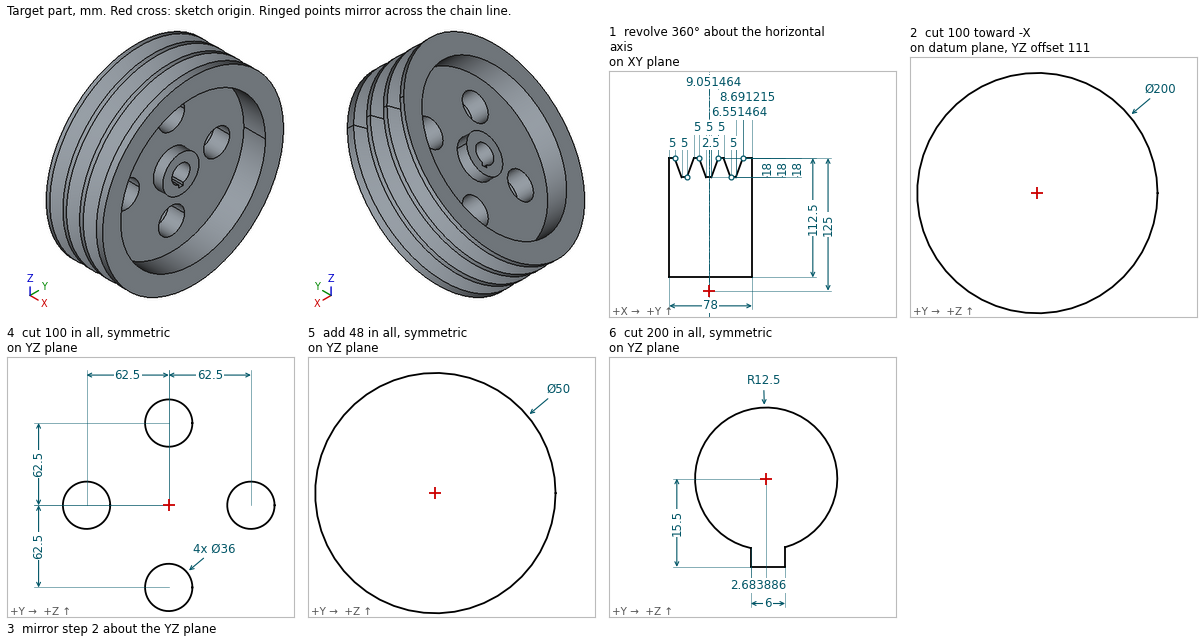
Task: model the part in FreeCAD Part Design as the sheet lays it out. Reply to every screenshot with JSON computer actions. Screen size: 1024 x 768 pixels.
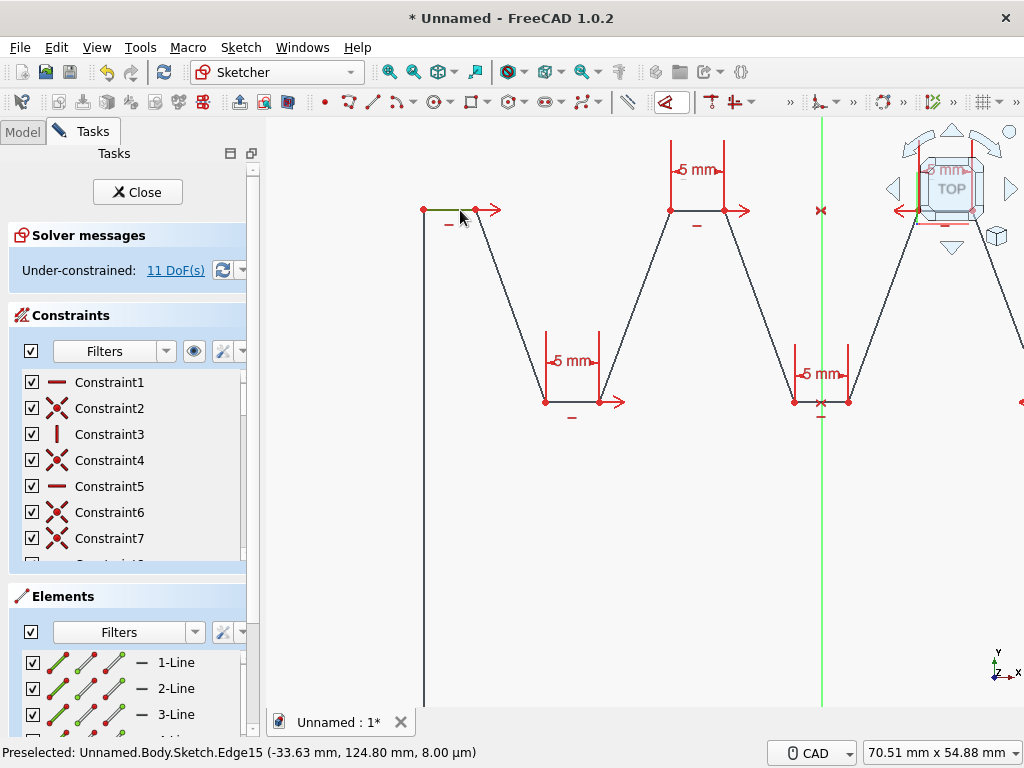
{"action": "left_click", "coordinate": [684, 102]}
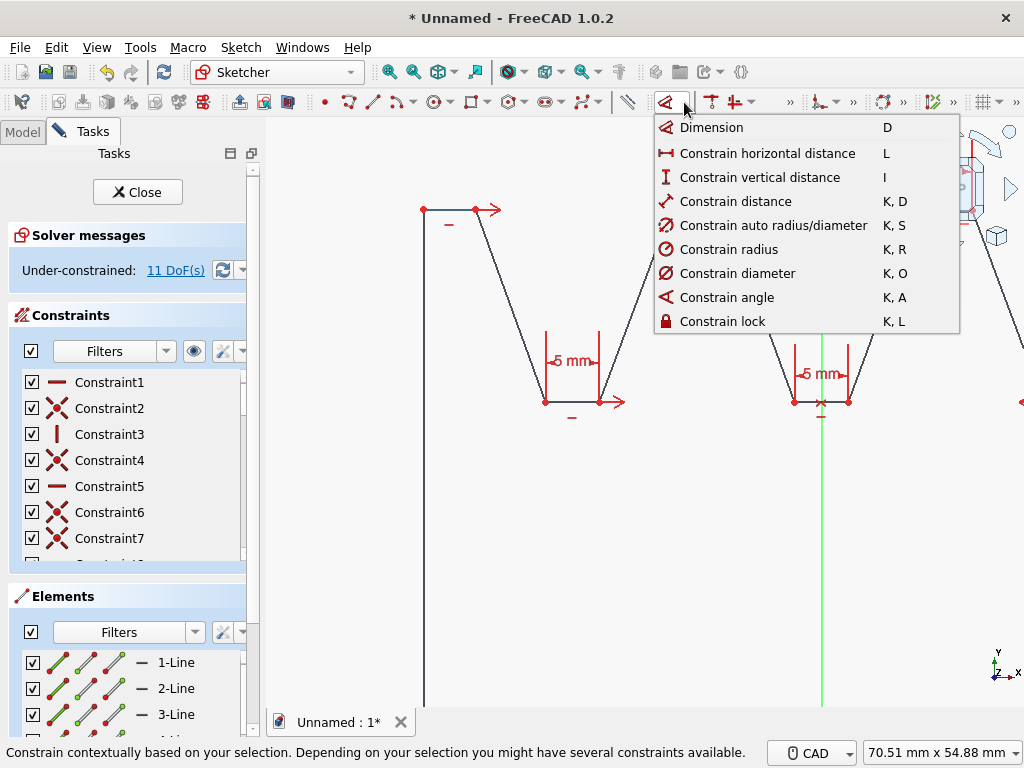
{"action": "left_click", "coordinate": [807, 153]}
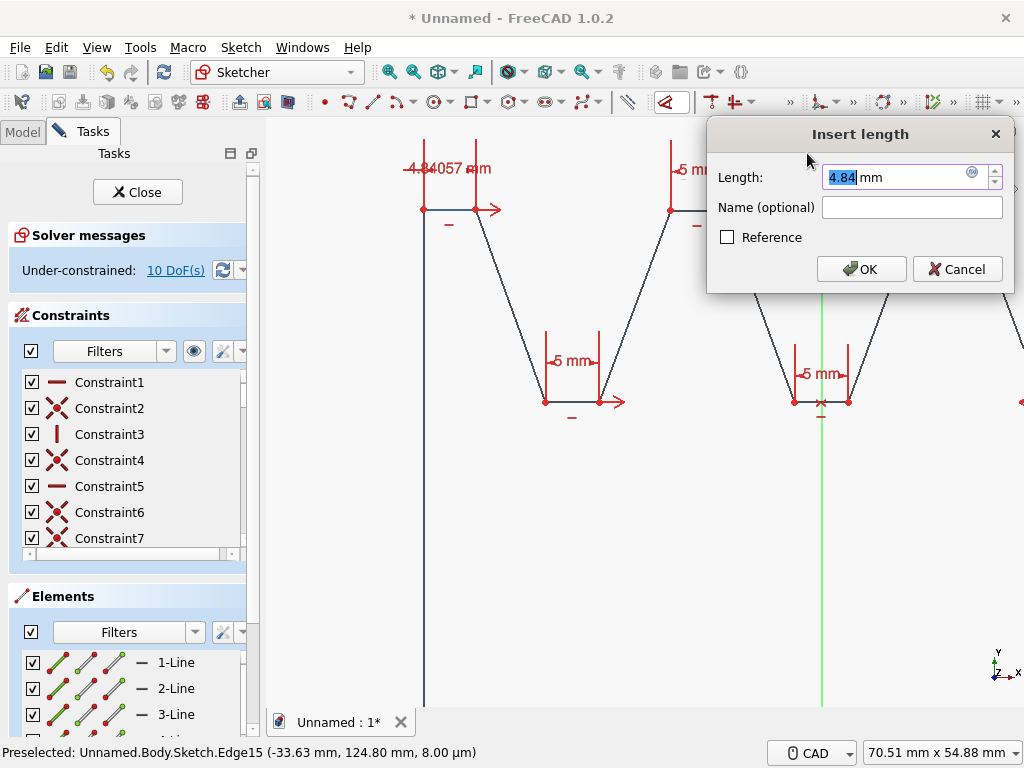
{"action": "type", "text": "5"}
{"action": "key", "text": "Return"}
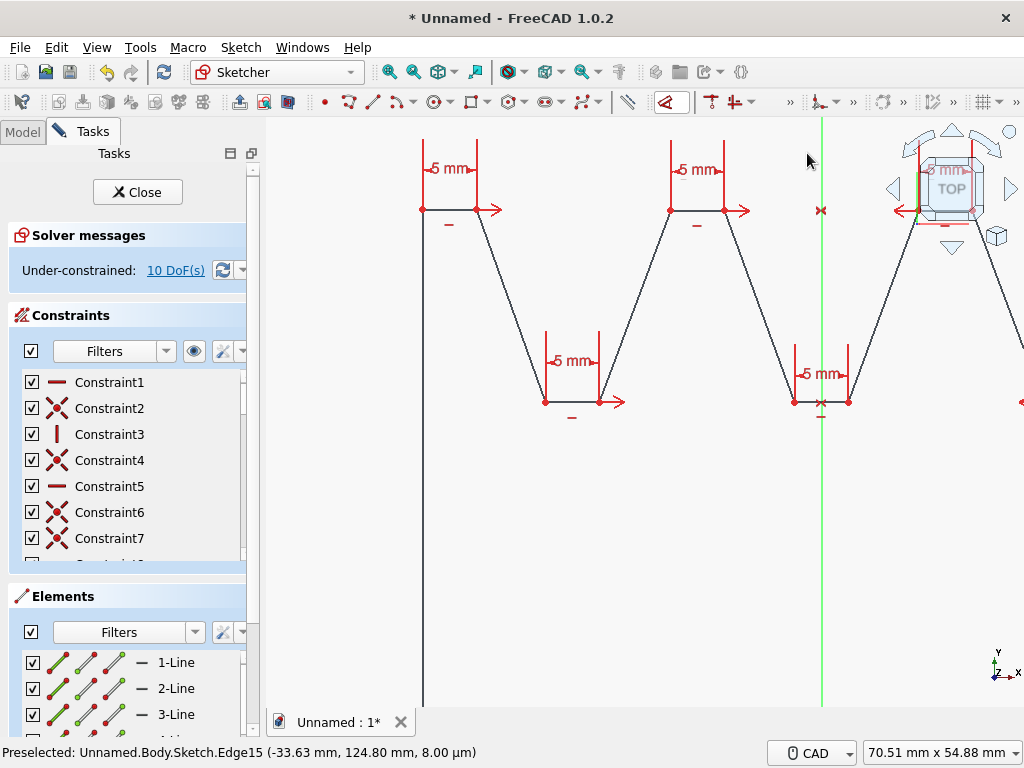
{"action": "scroll", "coordinate": [462, 210], "scroll_direction": "down", "scroll_amount": 6}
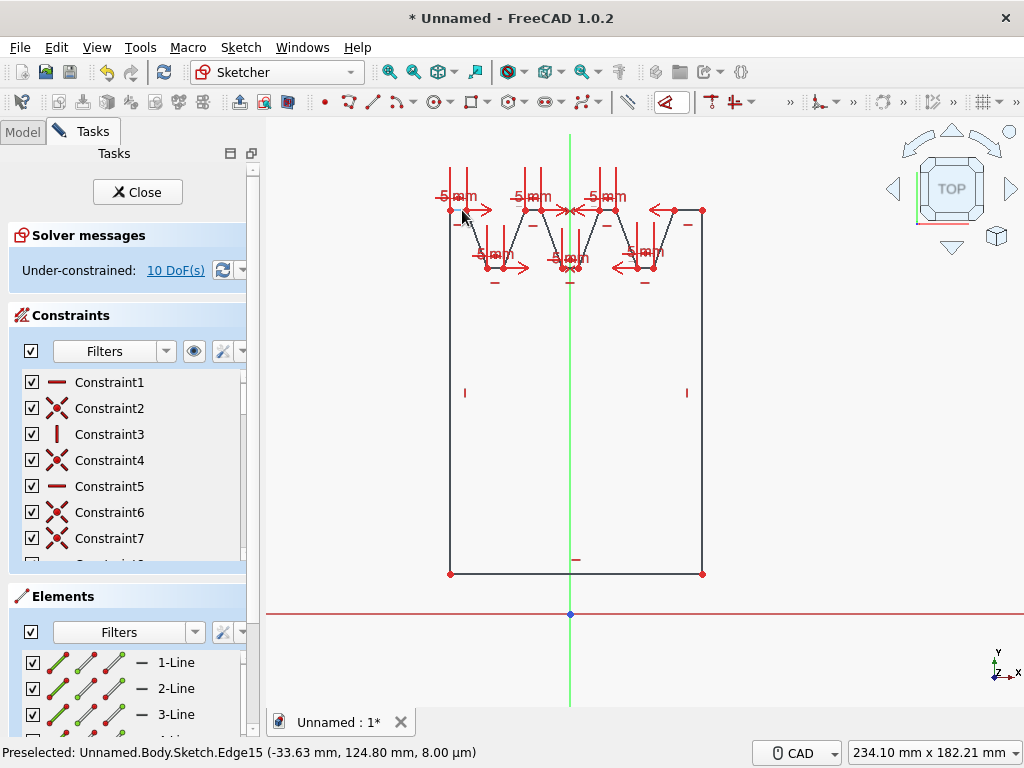
{"action": "left_click", "coordinate": [526, 574]}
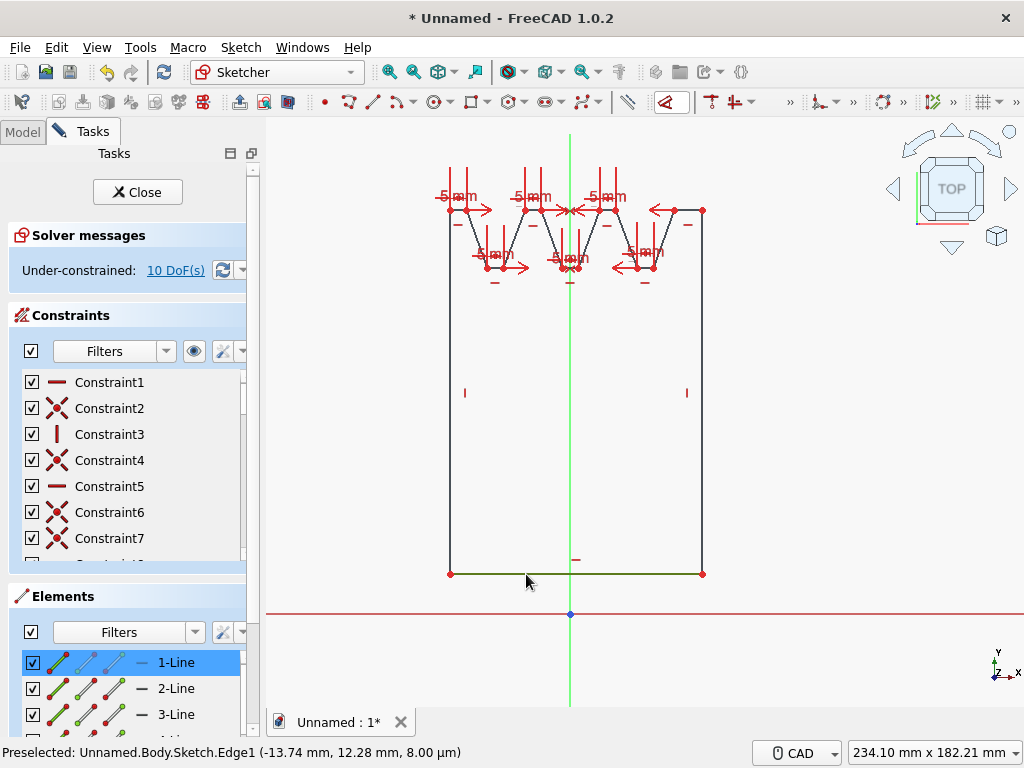
{"action": "key", "text": "l"}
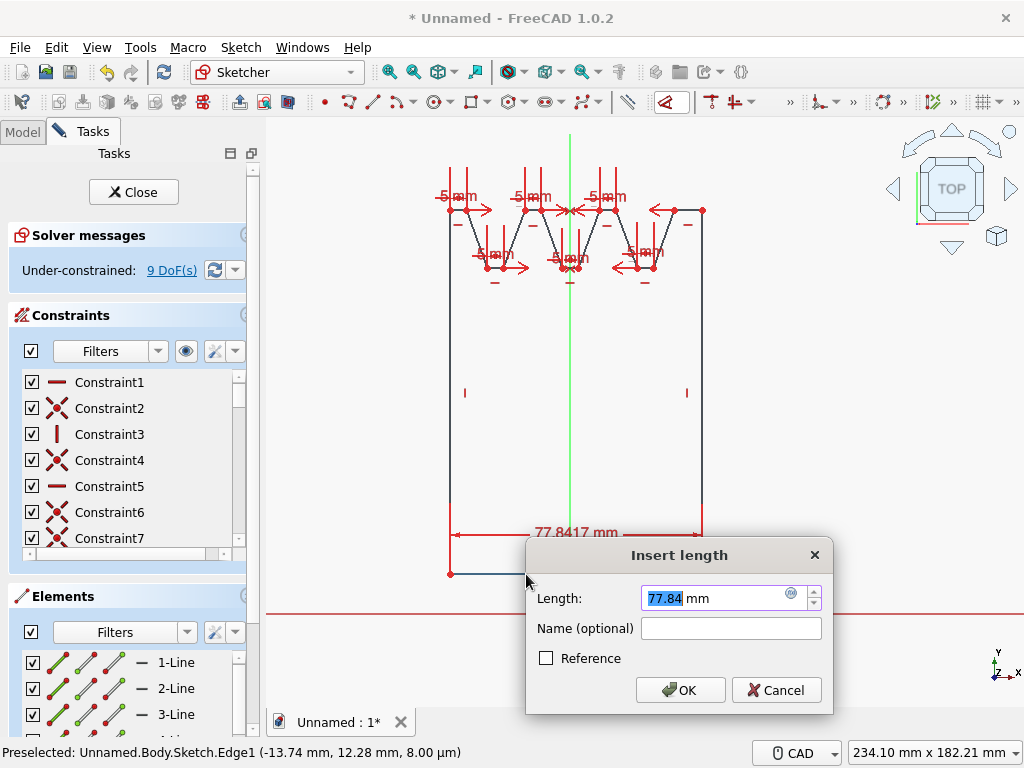
{"action": "type", "text": "78"}
{"action": "key", "text": "Return"}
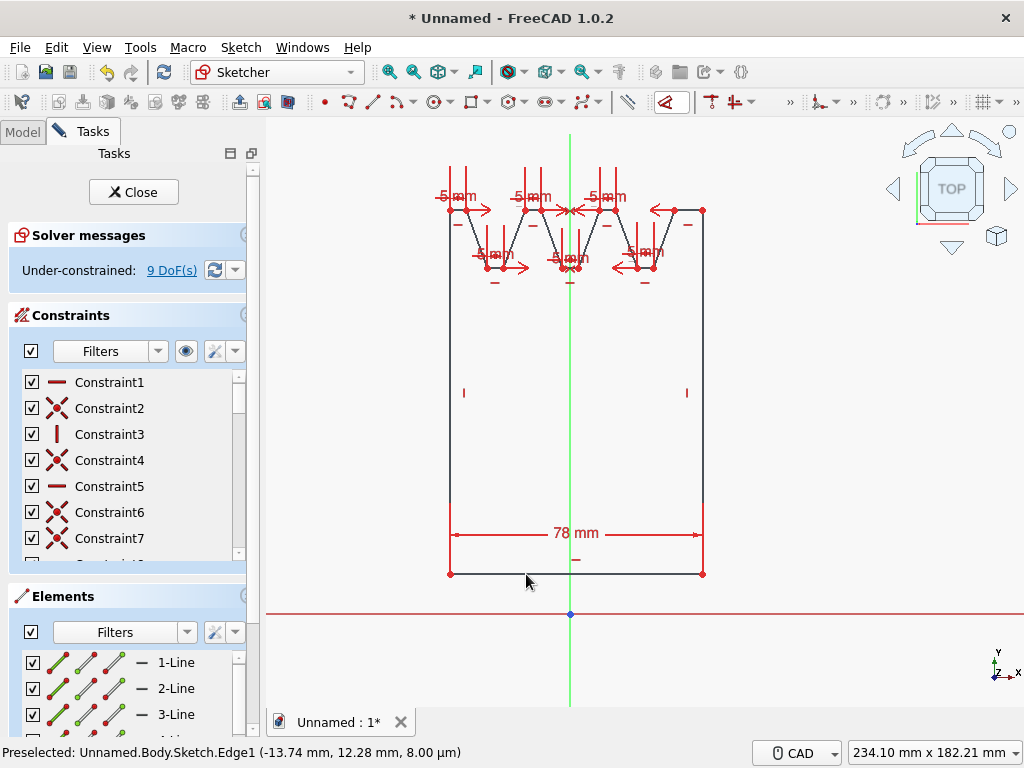
{"action": "left_click", "coordinate": [668, 227]}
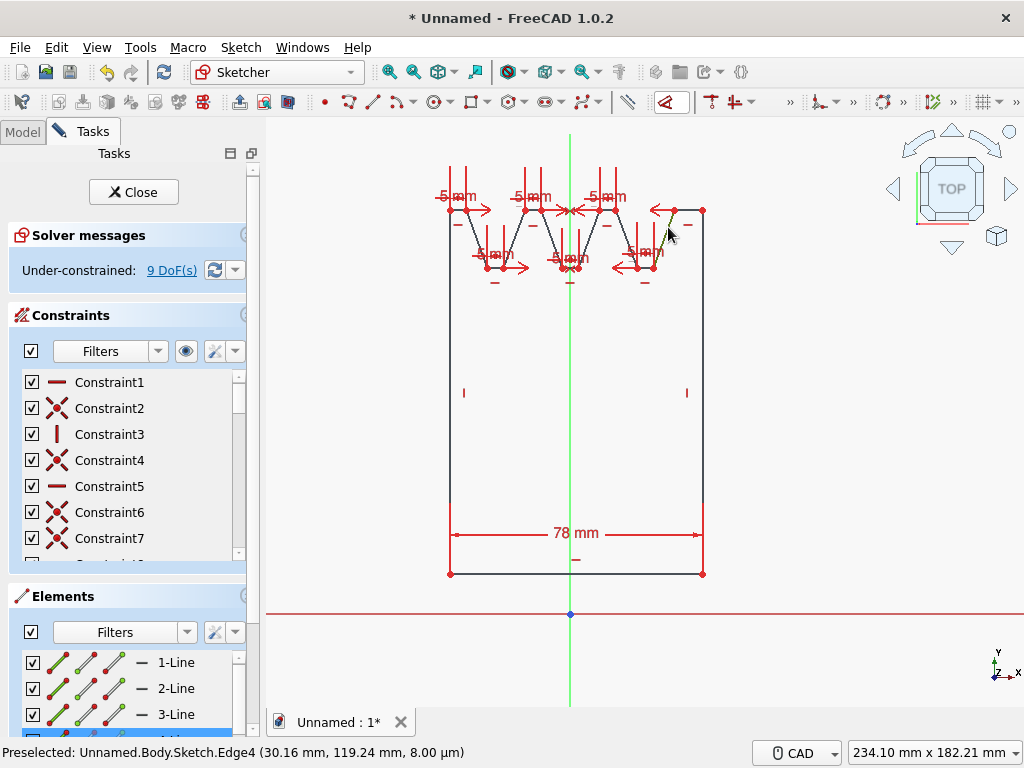
{"action": "key", "text": "i"}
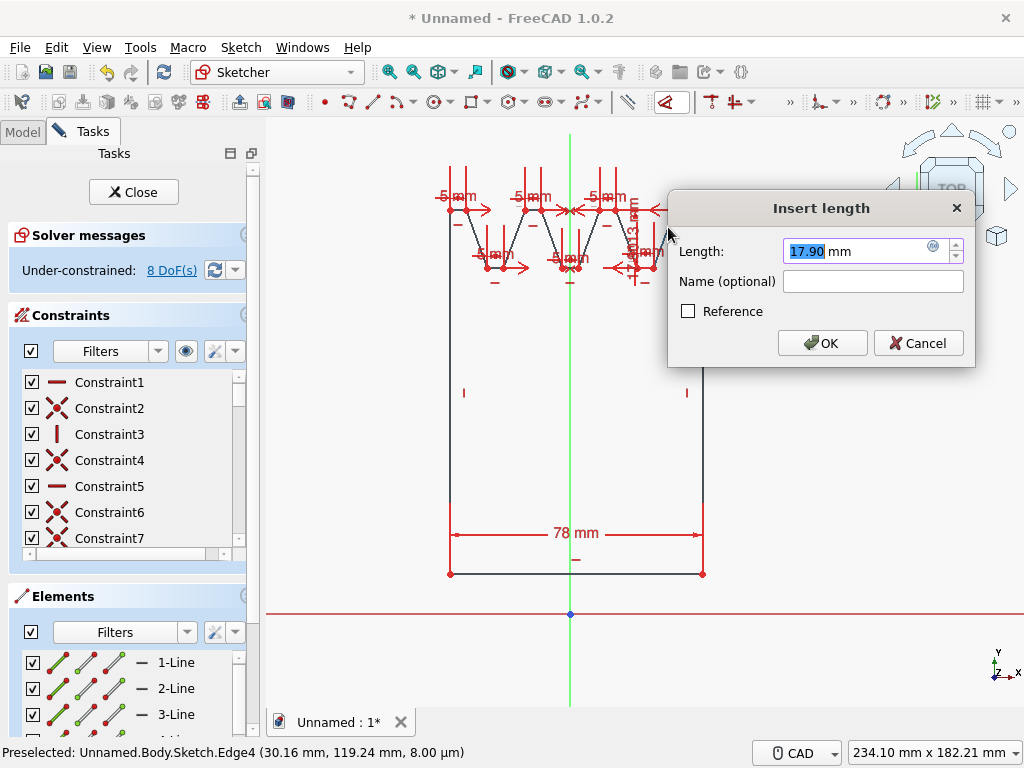
{"action": "type", "text": "18"}
{"action": "key", "text": "Return"}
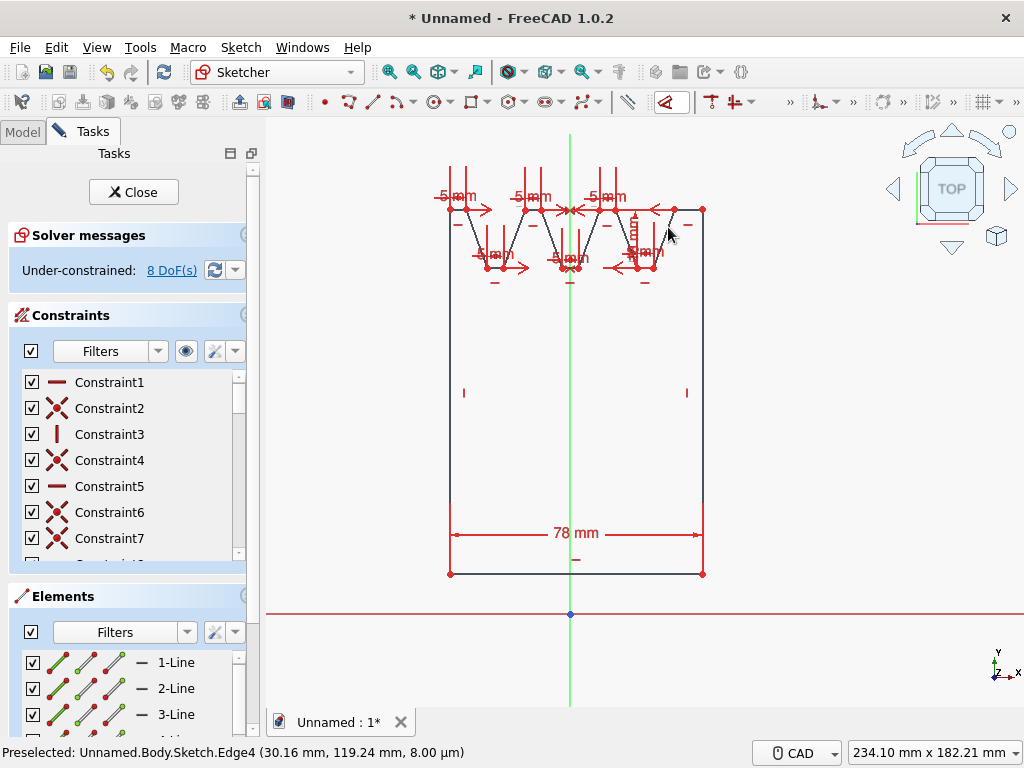
{"action": "left_click", "coordinate": [622, 228]}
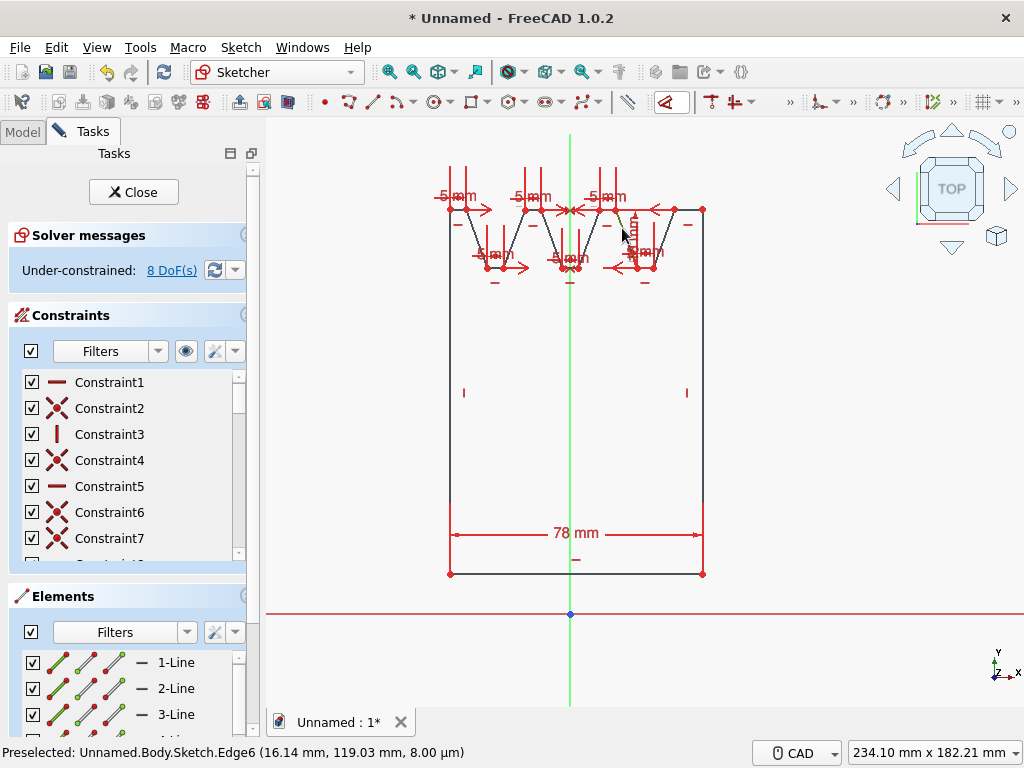
{"action": "left_click", "coordinate": [684, 102]}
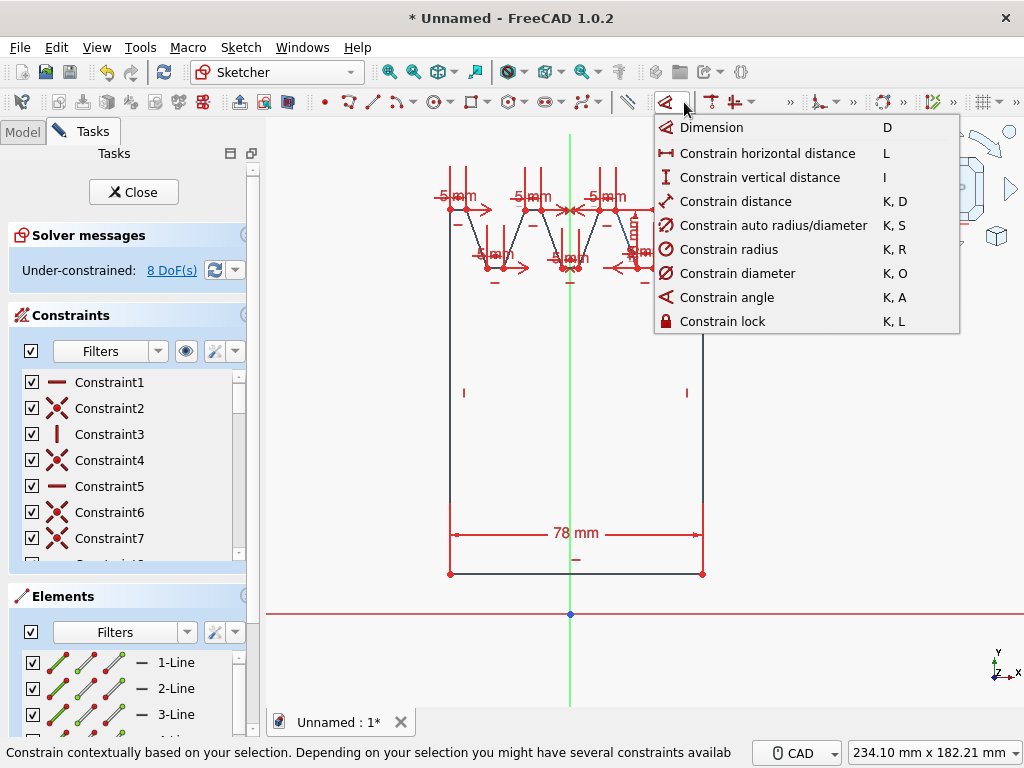
{"action": "left_click", "coordinate": [807, 177]}